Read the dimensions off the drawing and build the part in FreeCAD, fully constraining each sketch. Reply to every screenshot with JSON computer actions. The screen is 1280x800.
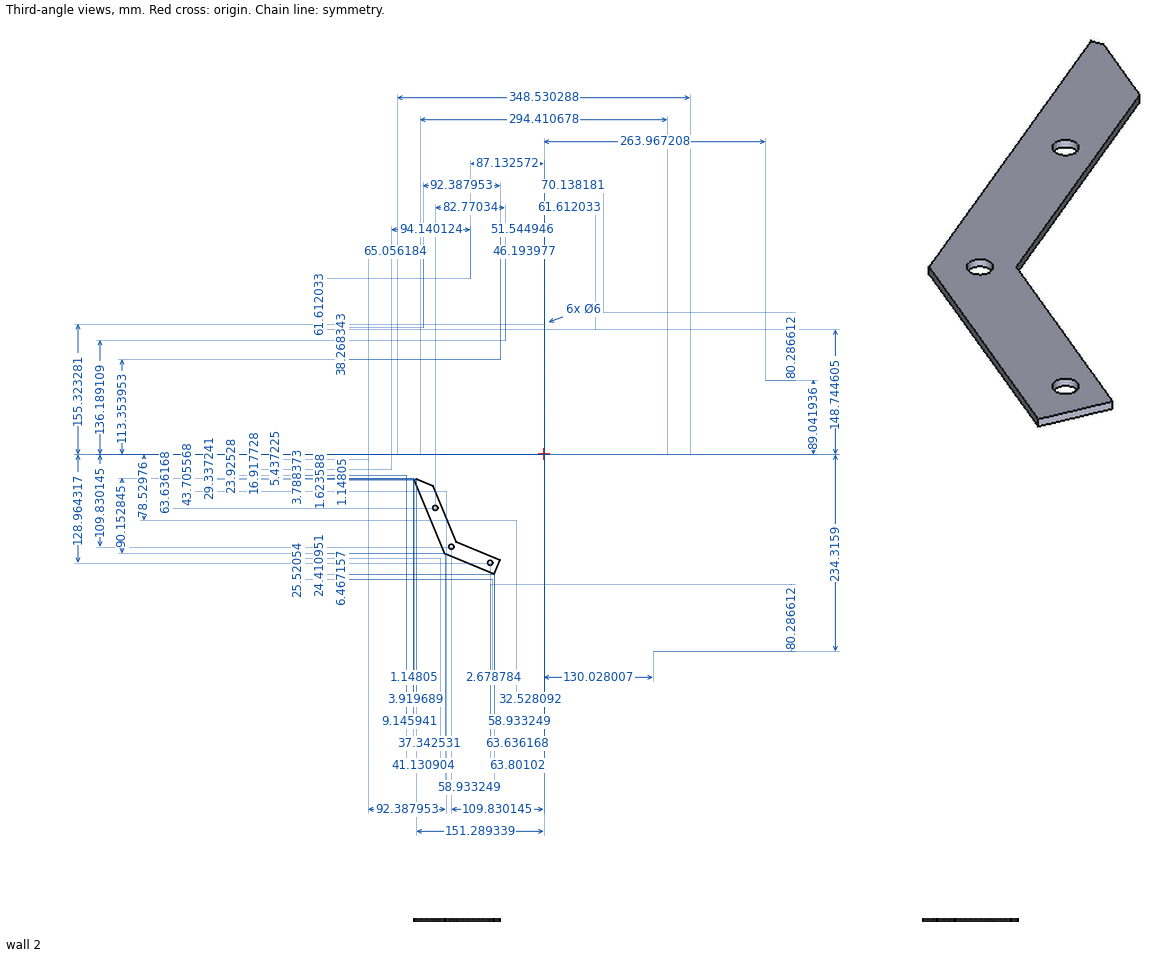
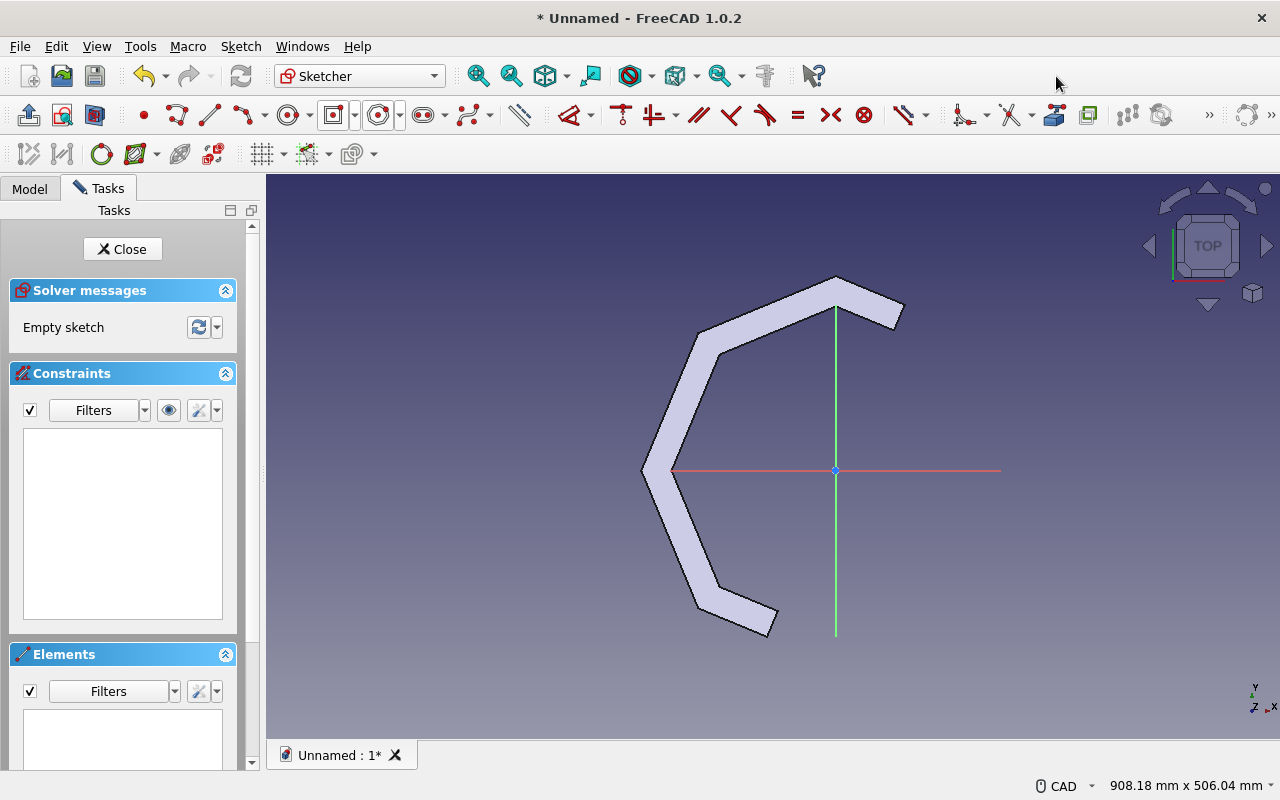
{"action": "scroll", "coordinate": [749, 317], "scroll_direction": "up", "scroll_amount": 2}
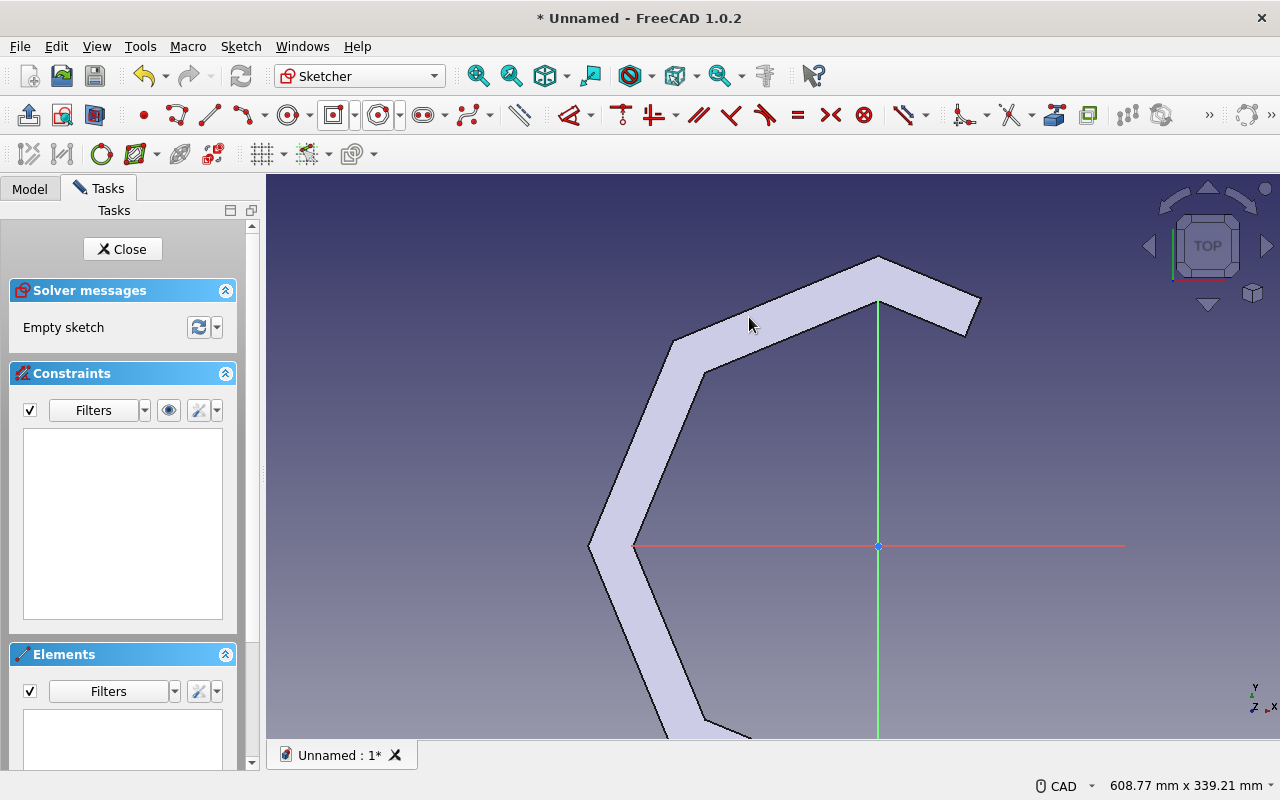
{"action": "left_click", "coordinate": [177, 116]}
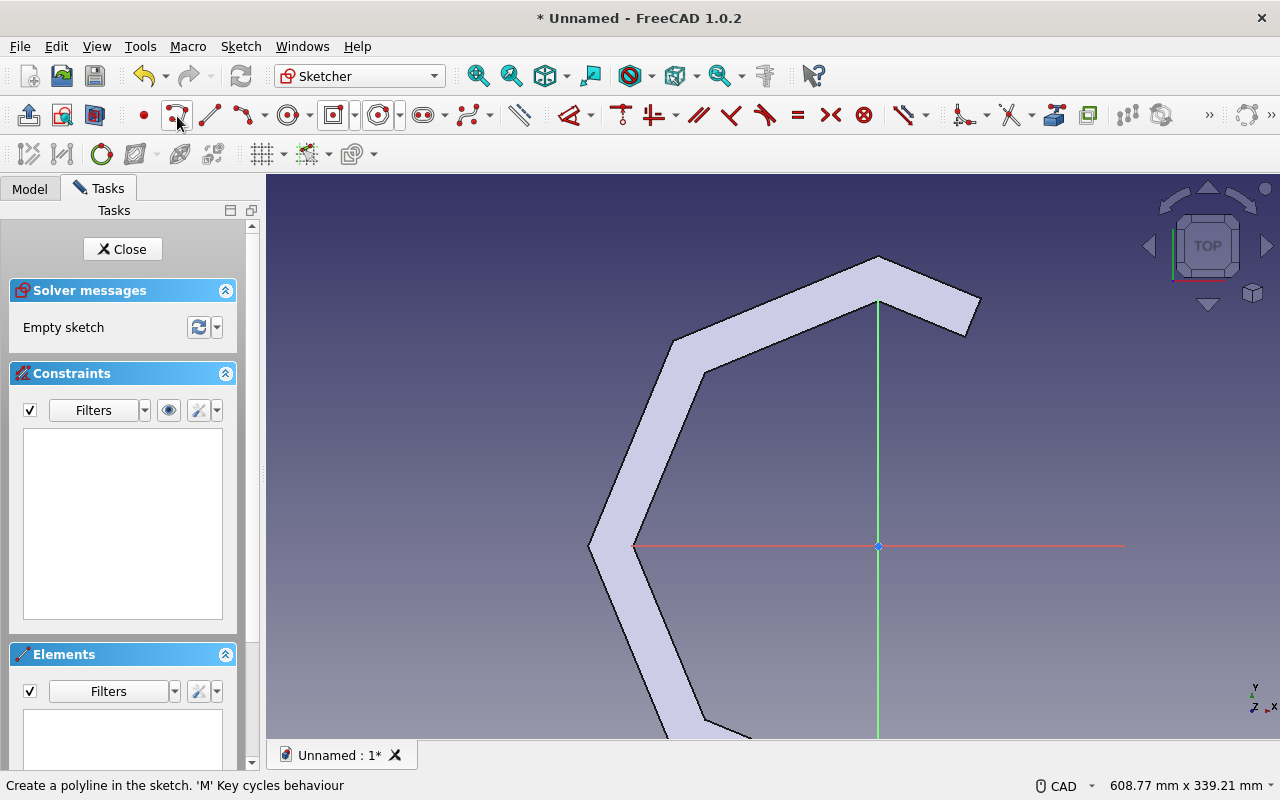
{"action": "left_click", "coordinate": [793, 357]}
{"action": "left_click", "coordinate": [639, 294]}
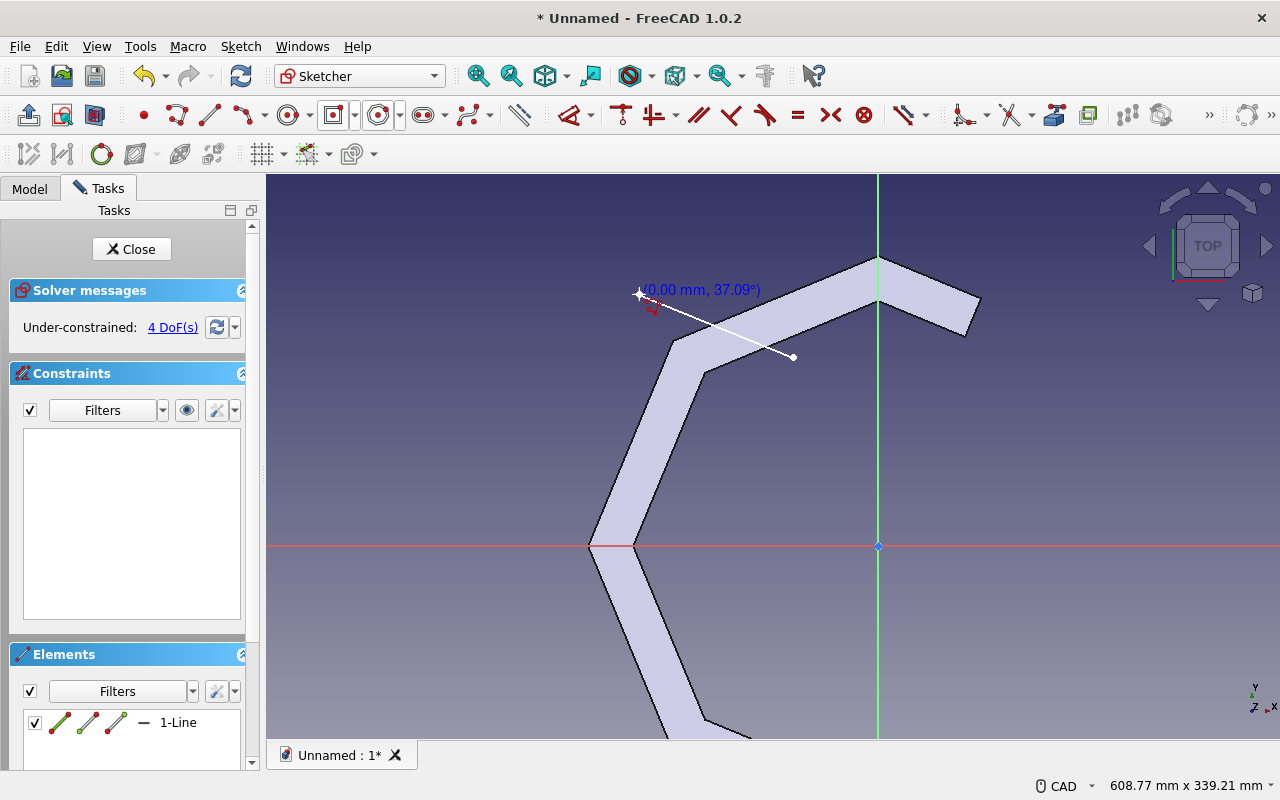
{"action": "scroll", "coordinate": [530, 555], "scroll_direction": "up", "scroll_amount": 3}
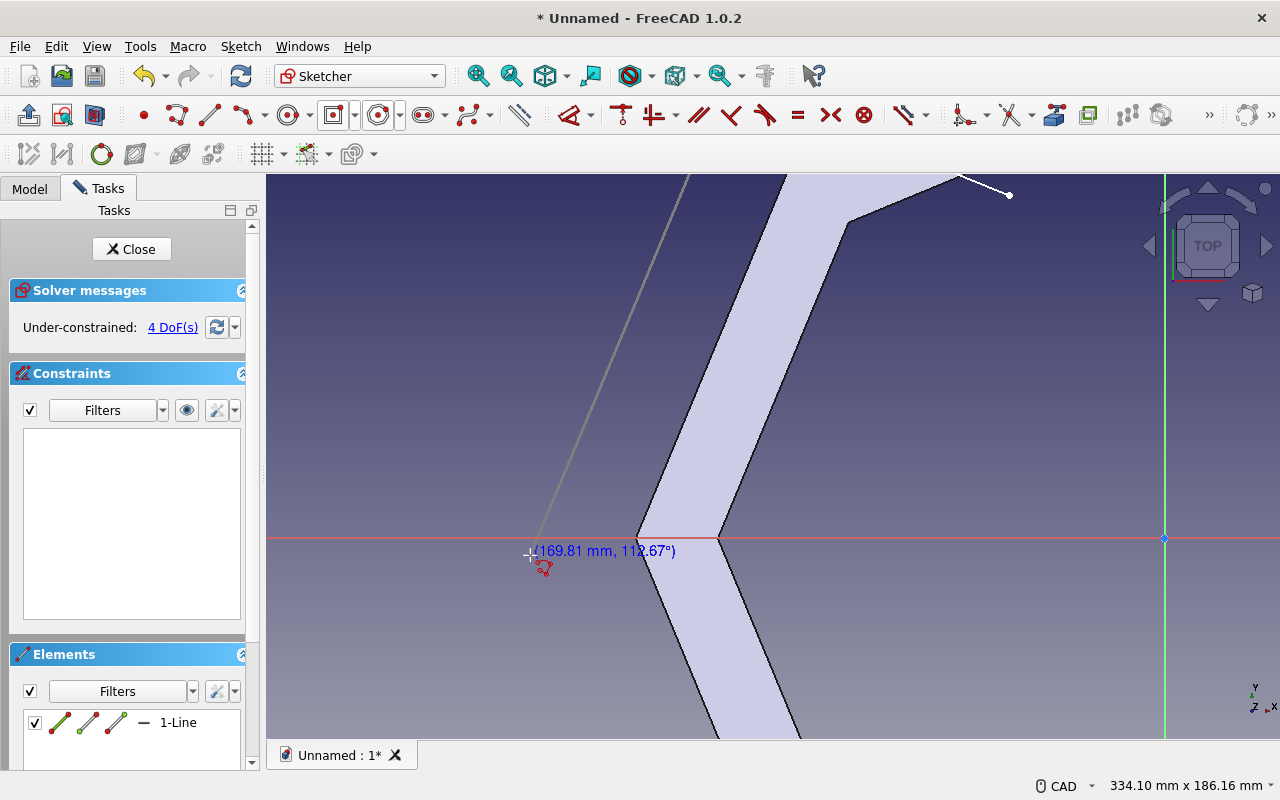
{"action": "left_click", "coordinate": [530, 555]}
{"action": "left_click", "coordinate": [811, 671]}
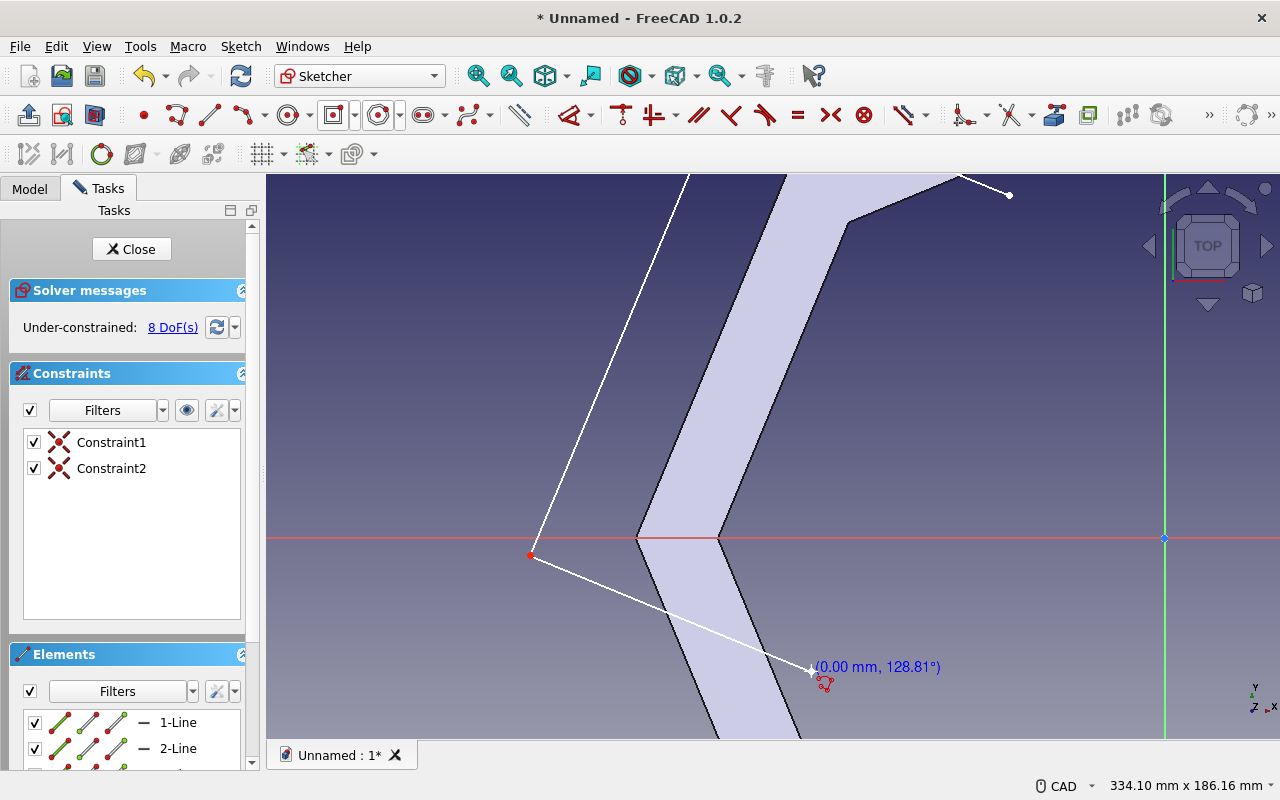
{"action": "scroll", "coordinate": [531, 556], "scroll_direction": "down", "scroll_amount": 3}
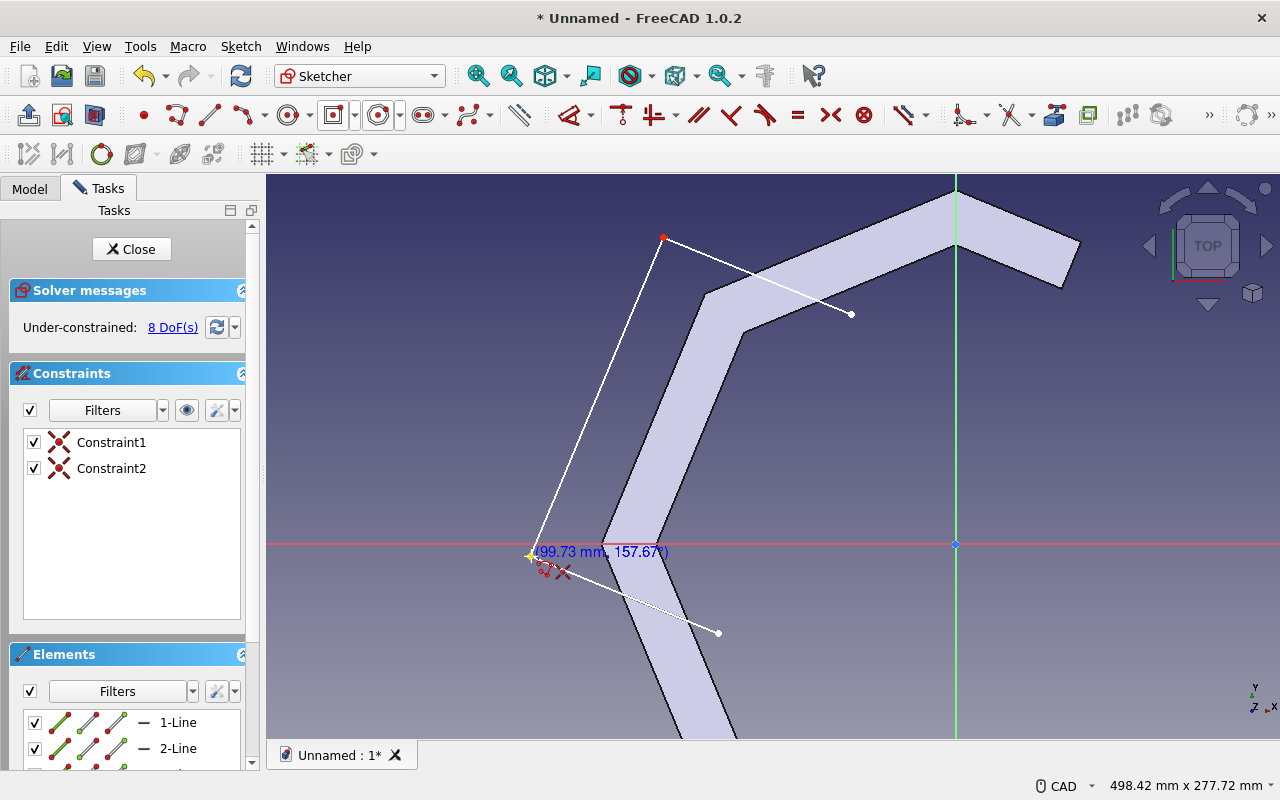
{"action": "left_click", "coordinate": [793, 358]}
{"action": "key", "text": "Escape"}
{"action": "key", "text": "Escape"}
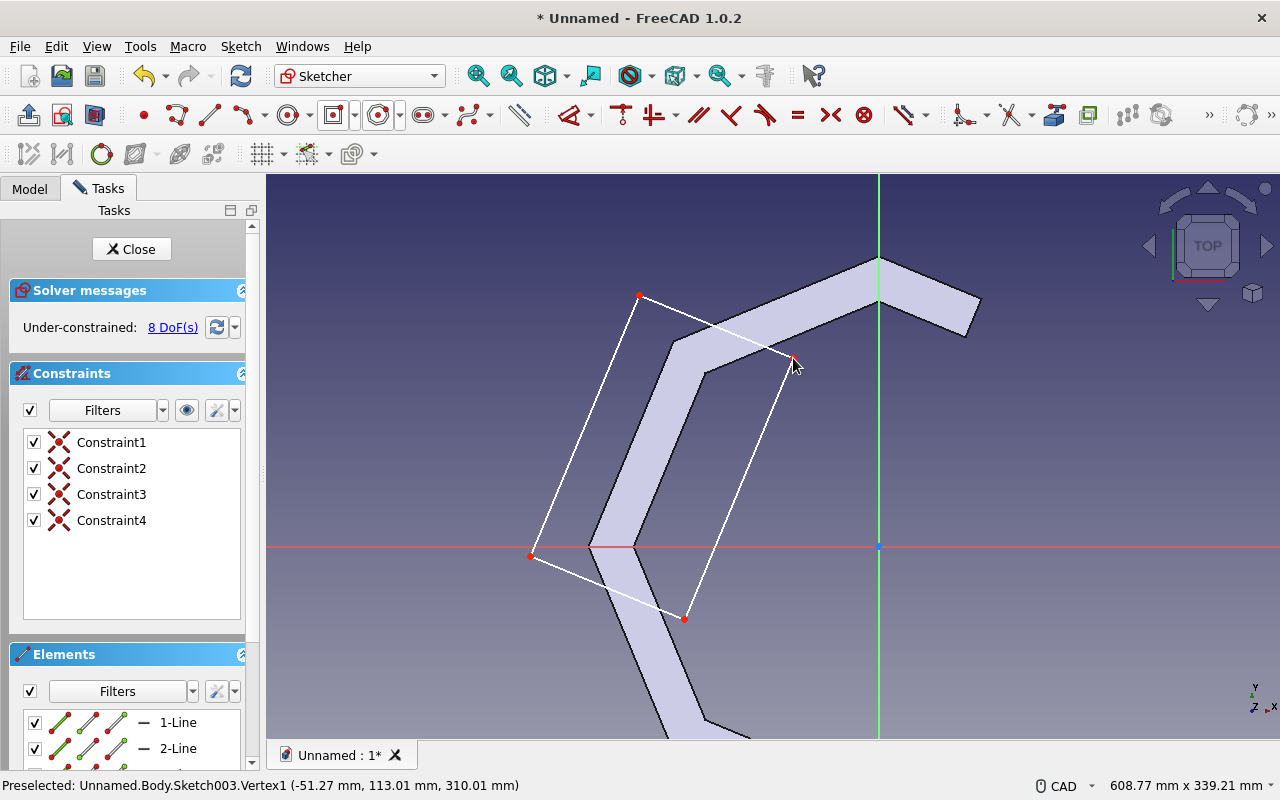
{"action": "left_click", "coordinate": [568, 116]}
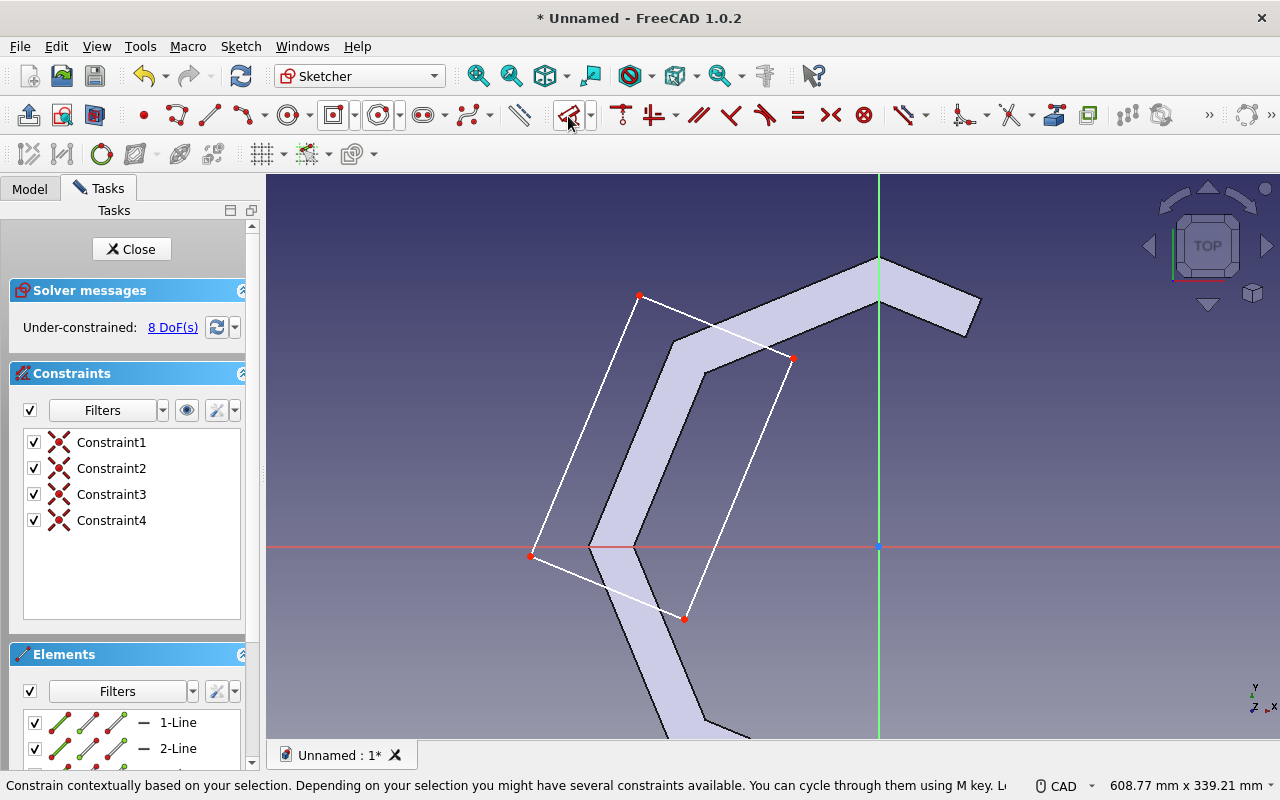
{"action": "scroll", "coordinate": [531, 556], "scroll_direction": "up", "scroll_amount": 8}